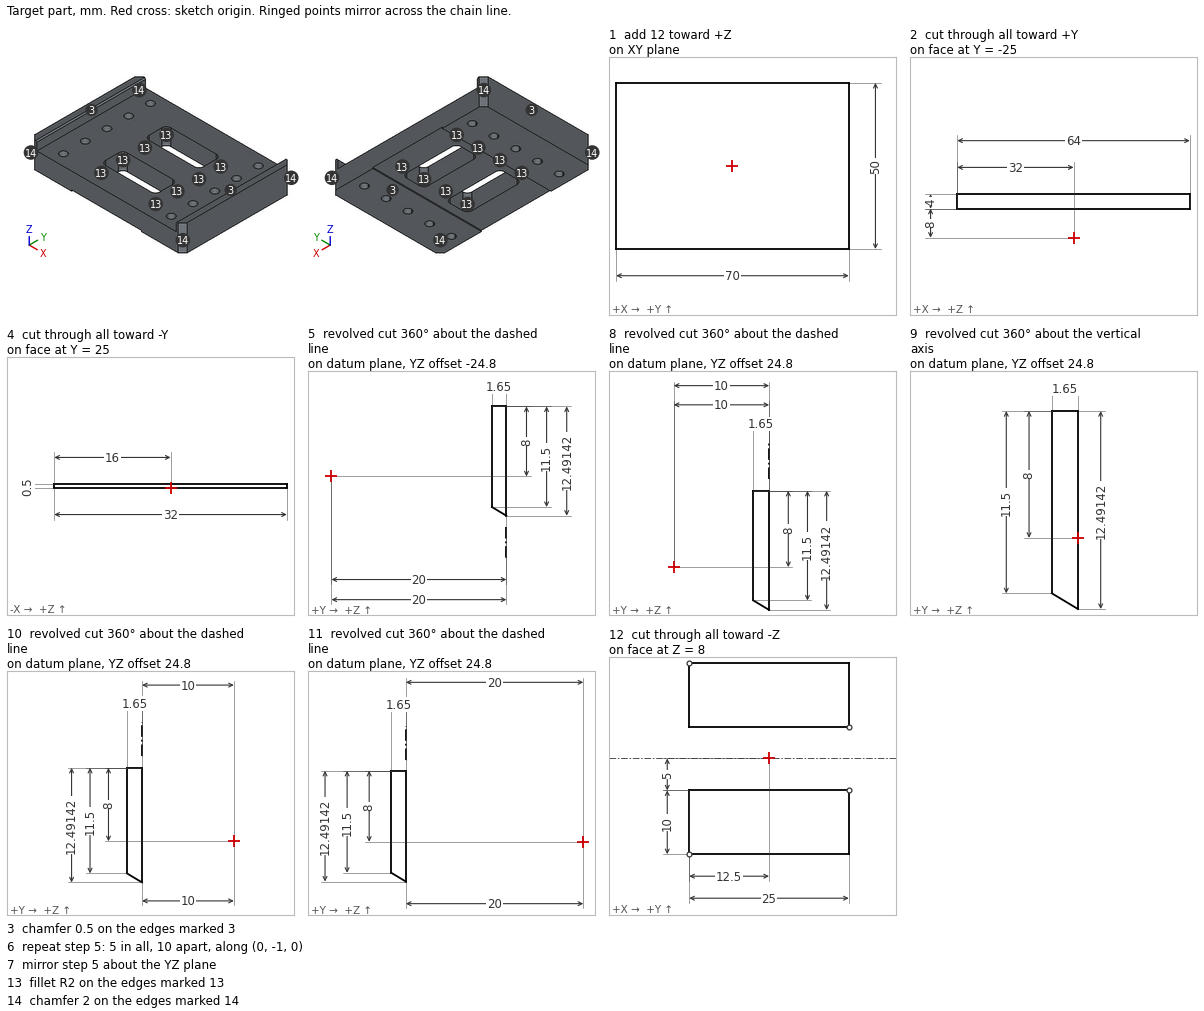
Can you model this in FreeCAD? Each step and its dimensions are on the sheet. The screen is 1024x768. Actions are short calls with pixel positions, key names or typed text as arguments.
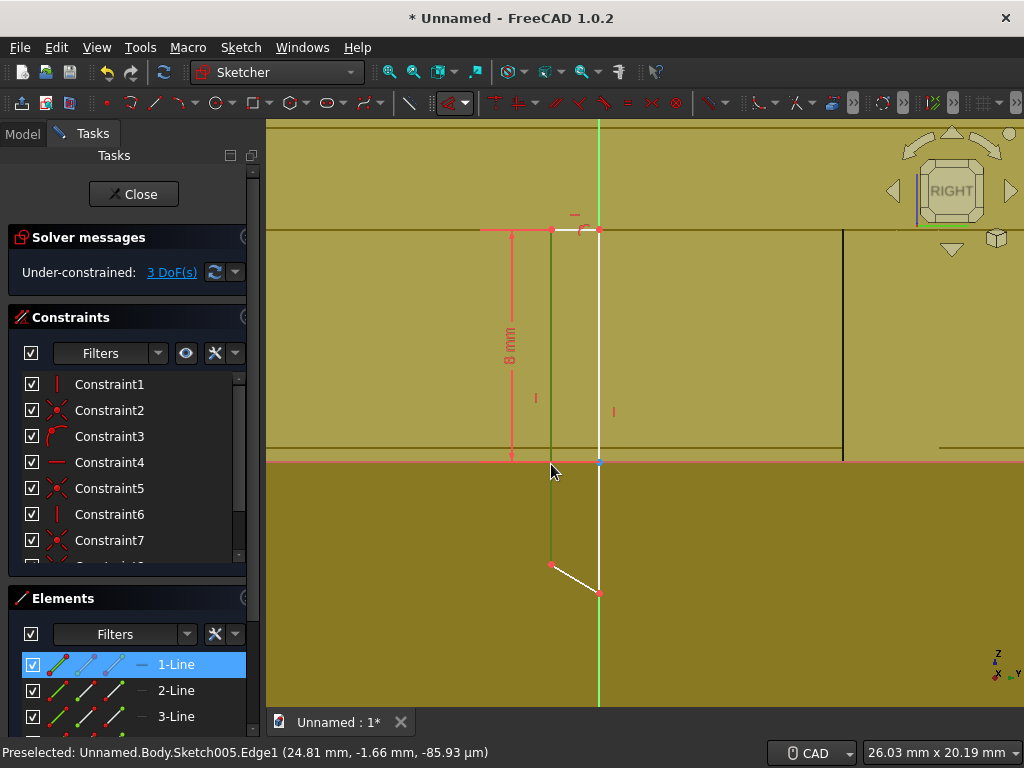
key(i)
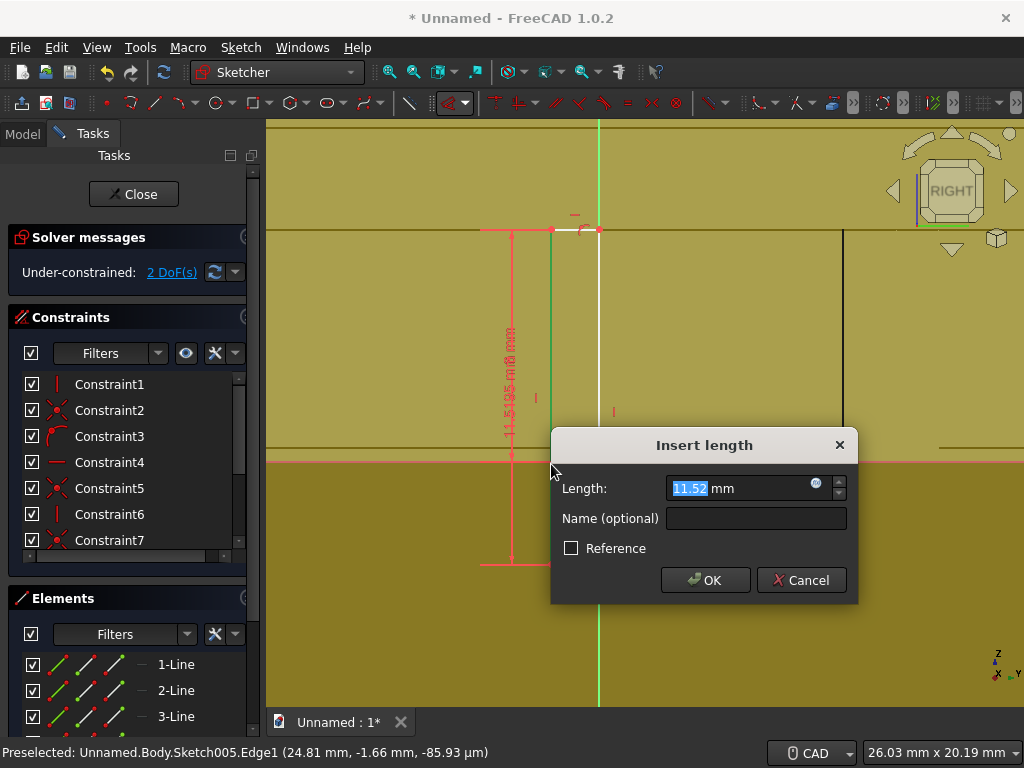
text(11.5)
key(Return)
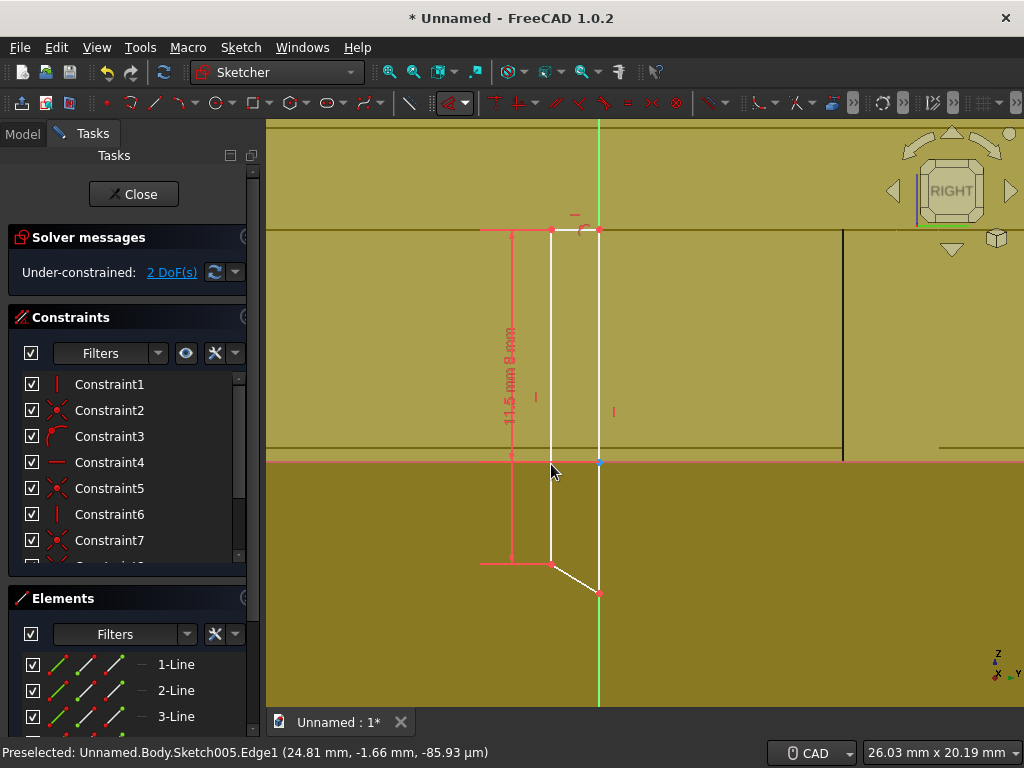
click(566, 230)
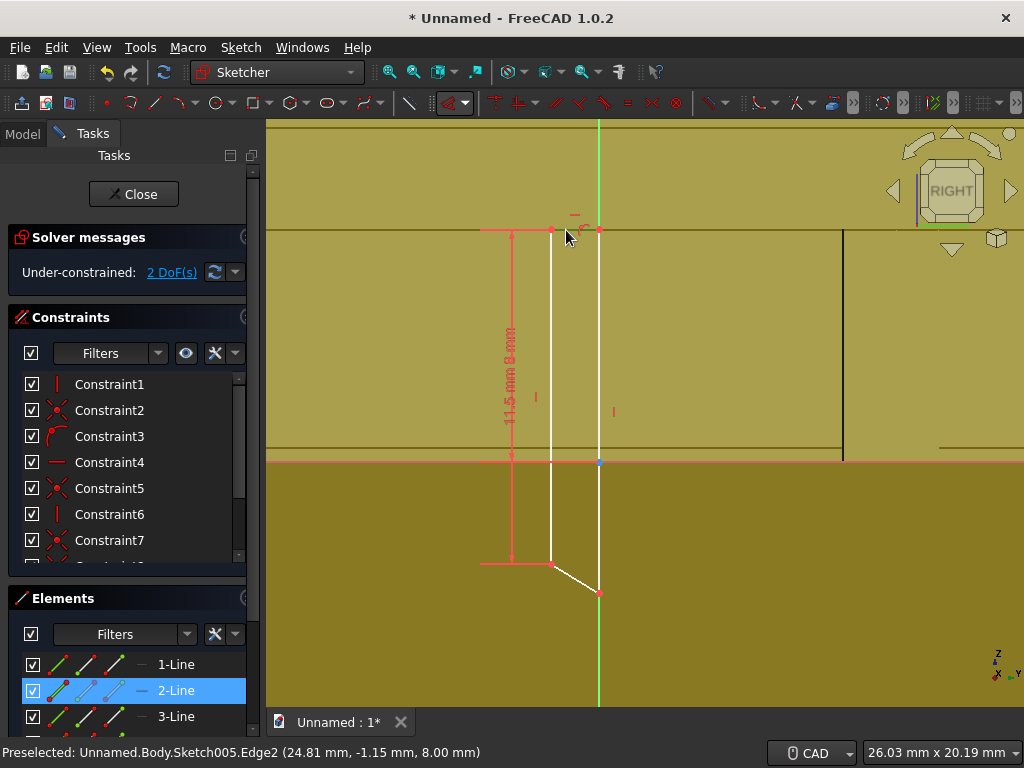
key(l)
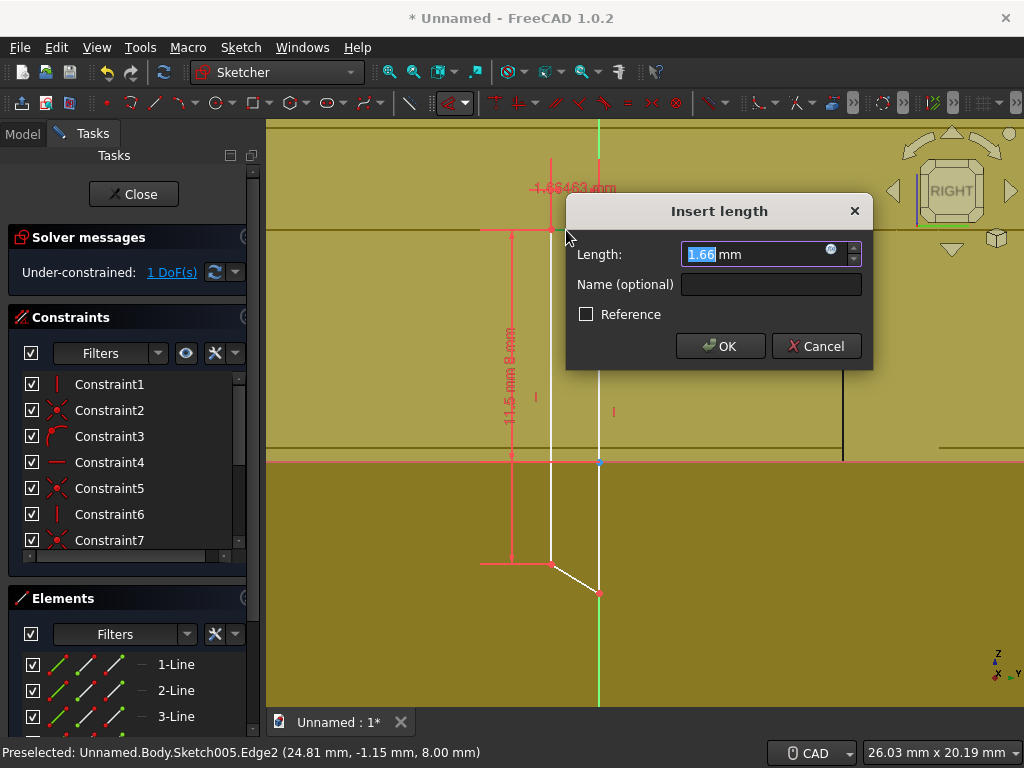
text(1.65)
key(Return)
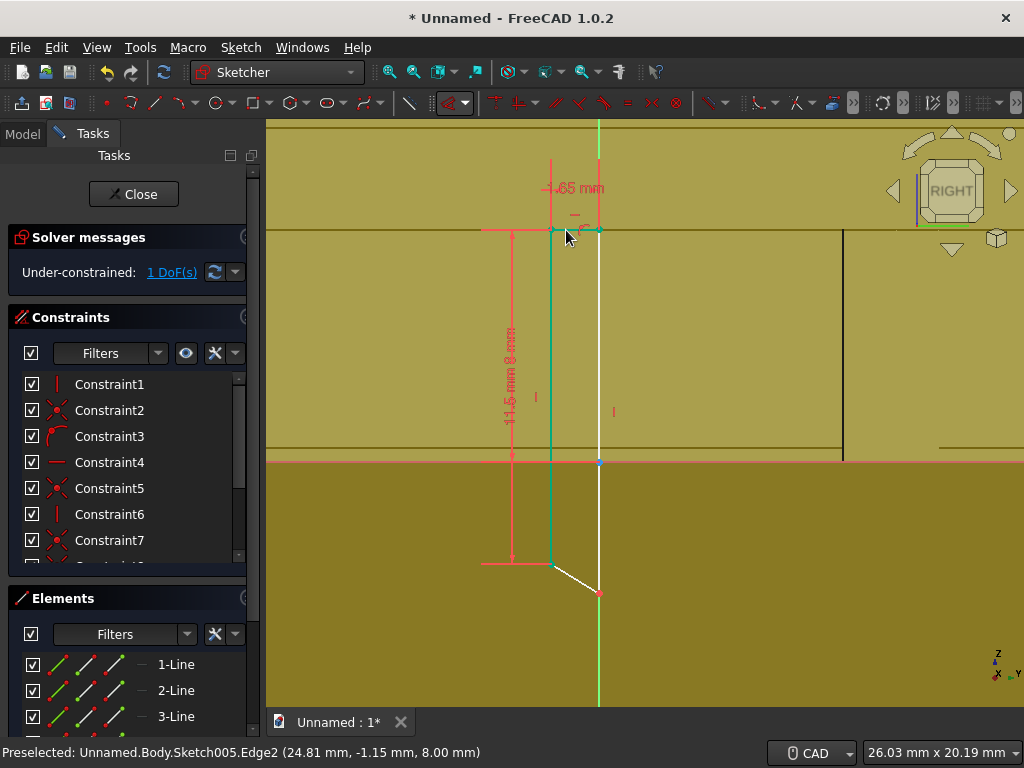
click(599, 339)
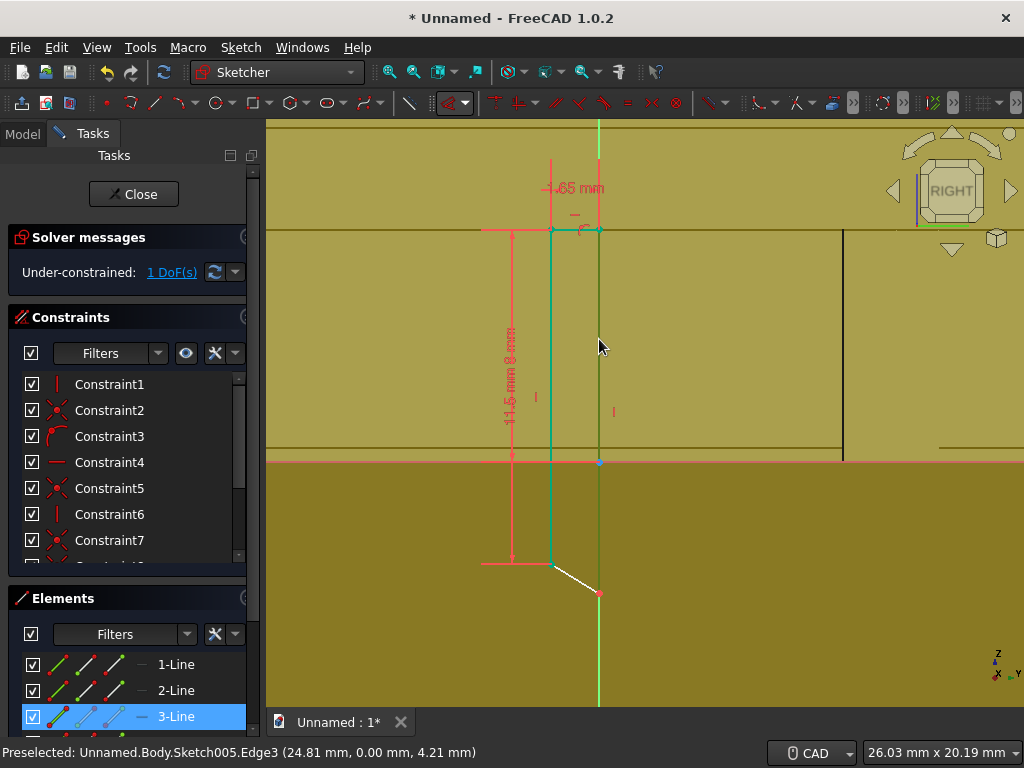
key(i)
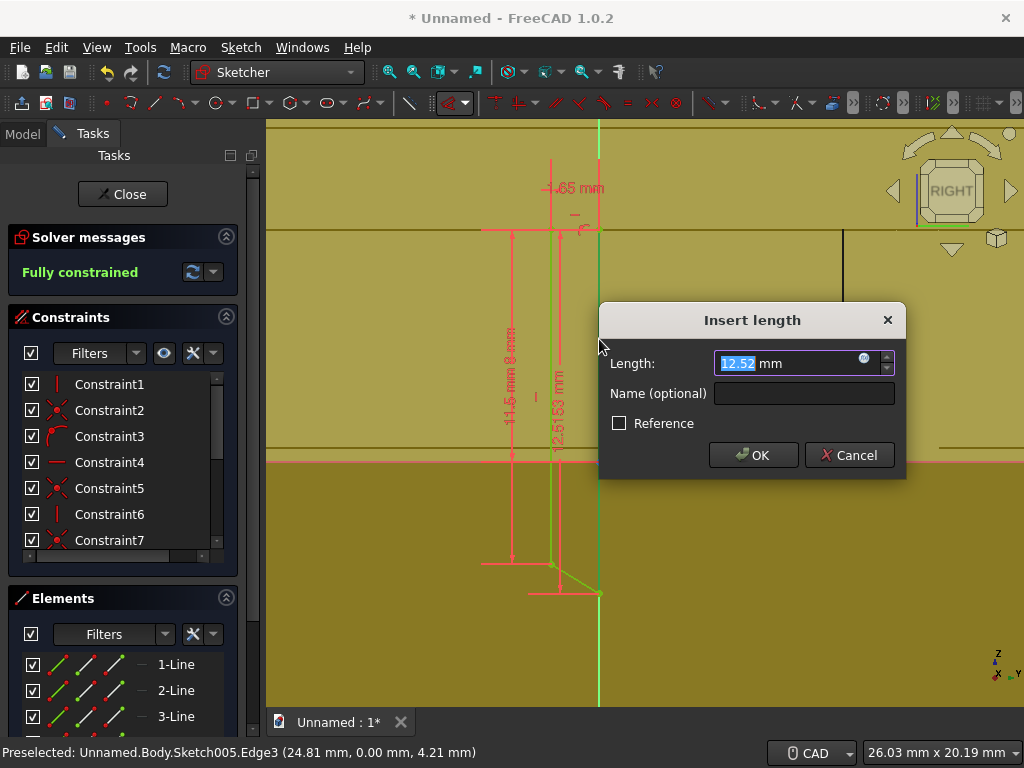
text(12.49142)
key(Return)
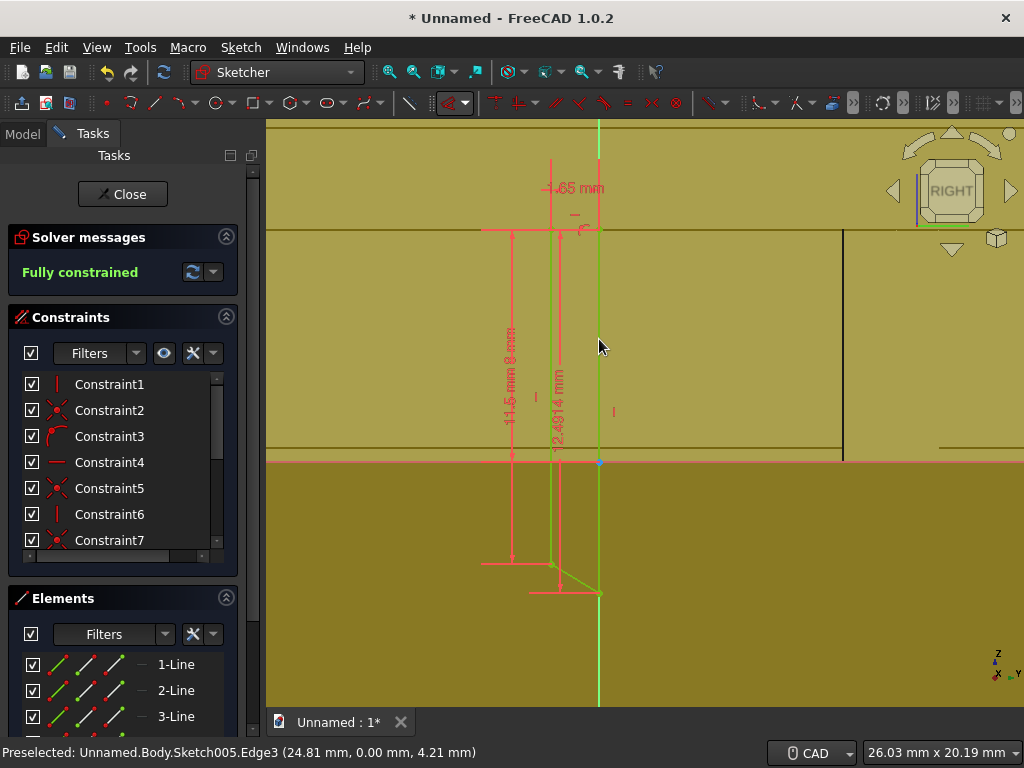
click(123, 194)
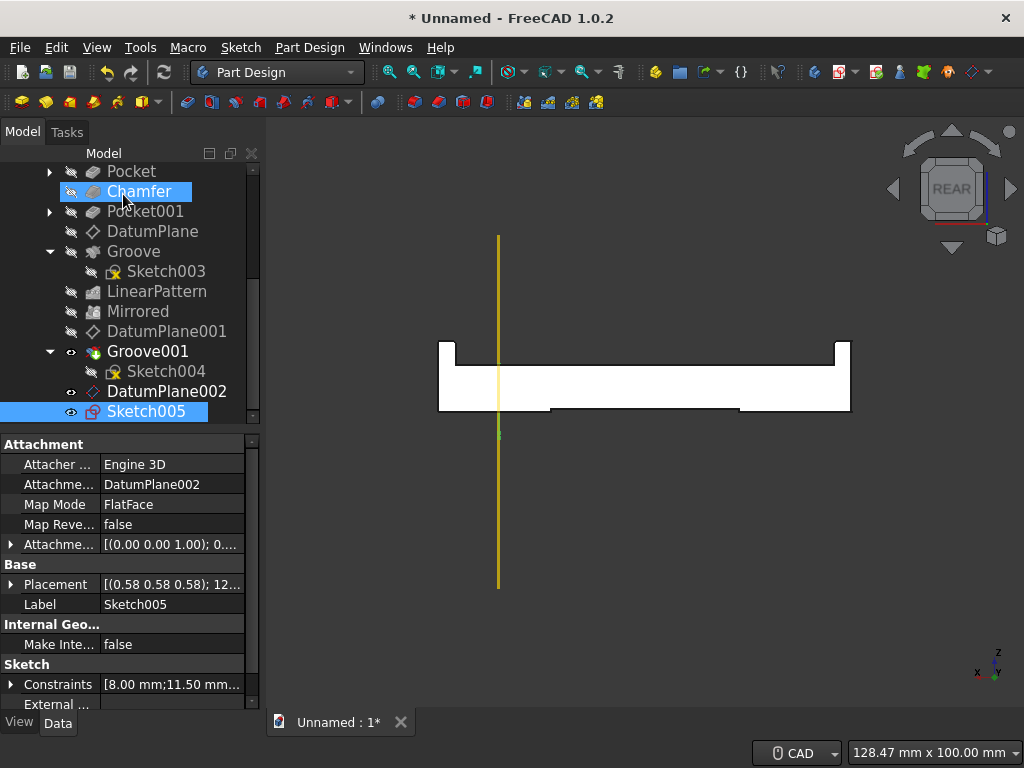
click(236, 102)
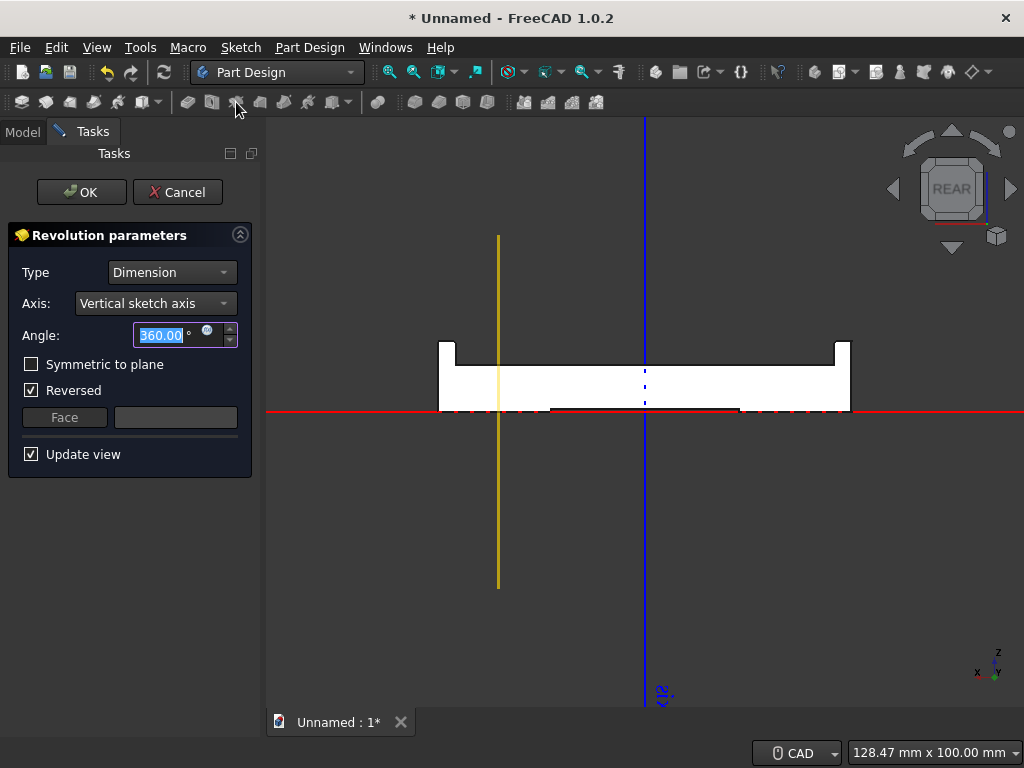
click(82, 192)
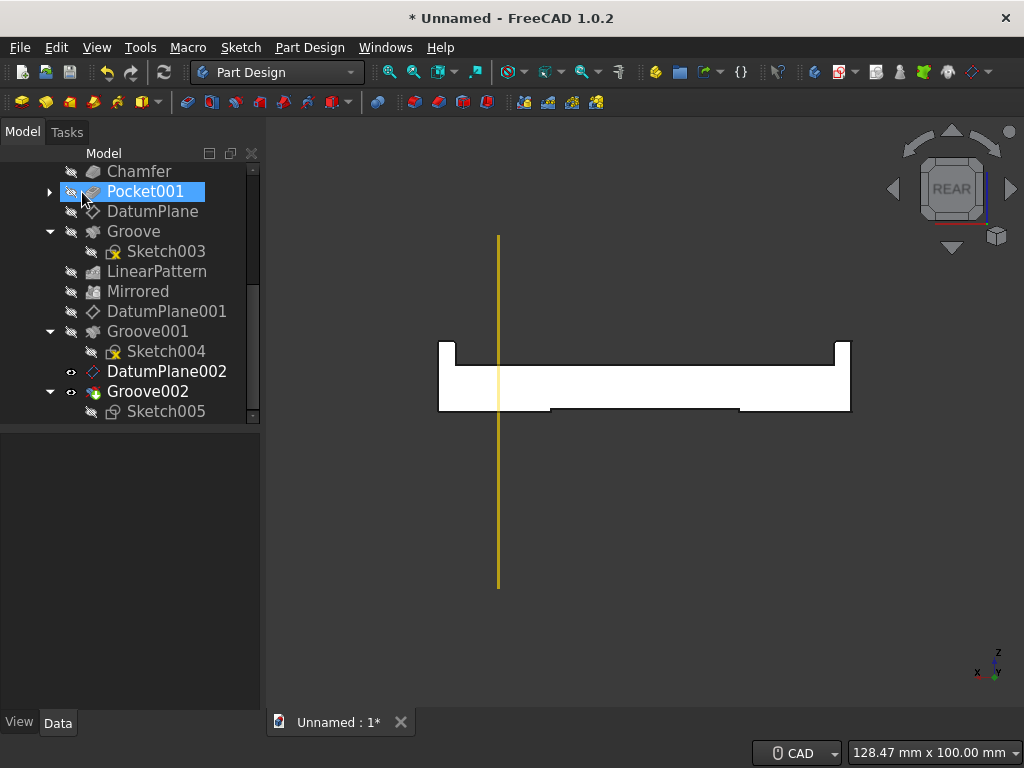
click(116, 372)
key(space)